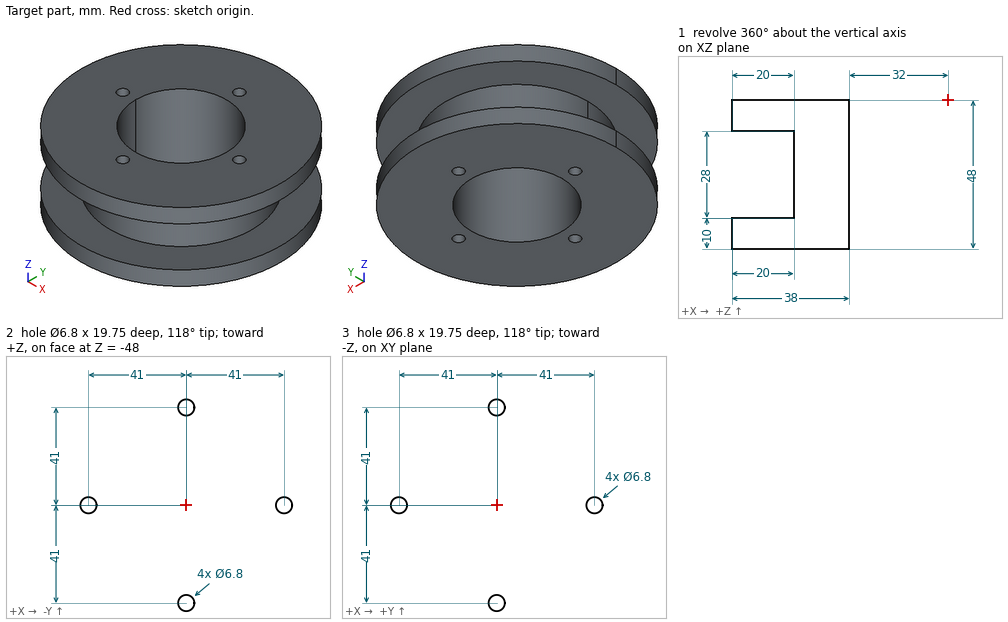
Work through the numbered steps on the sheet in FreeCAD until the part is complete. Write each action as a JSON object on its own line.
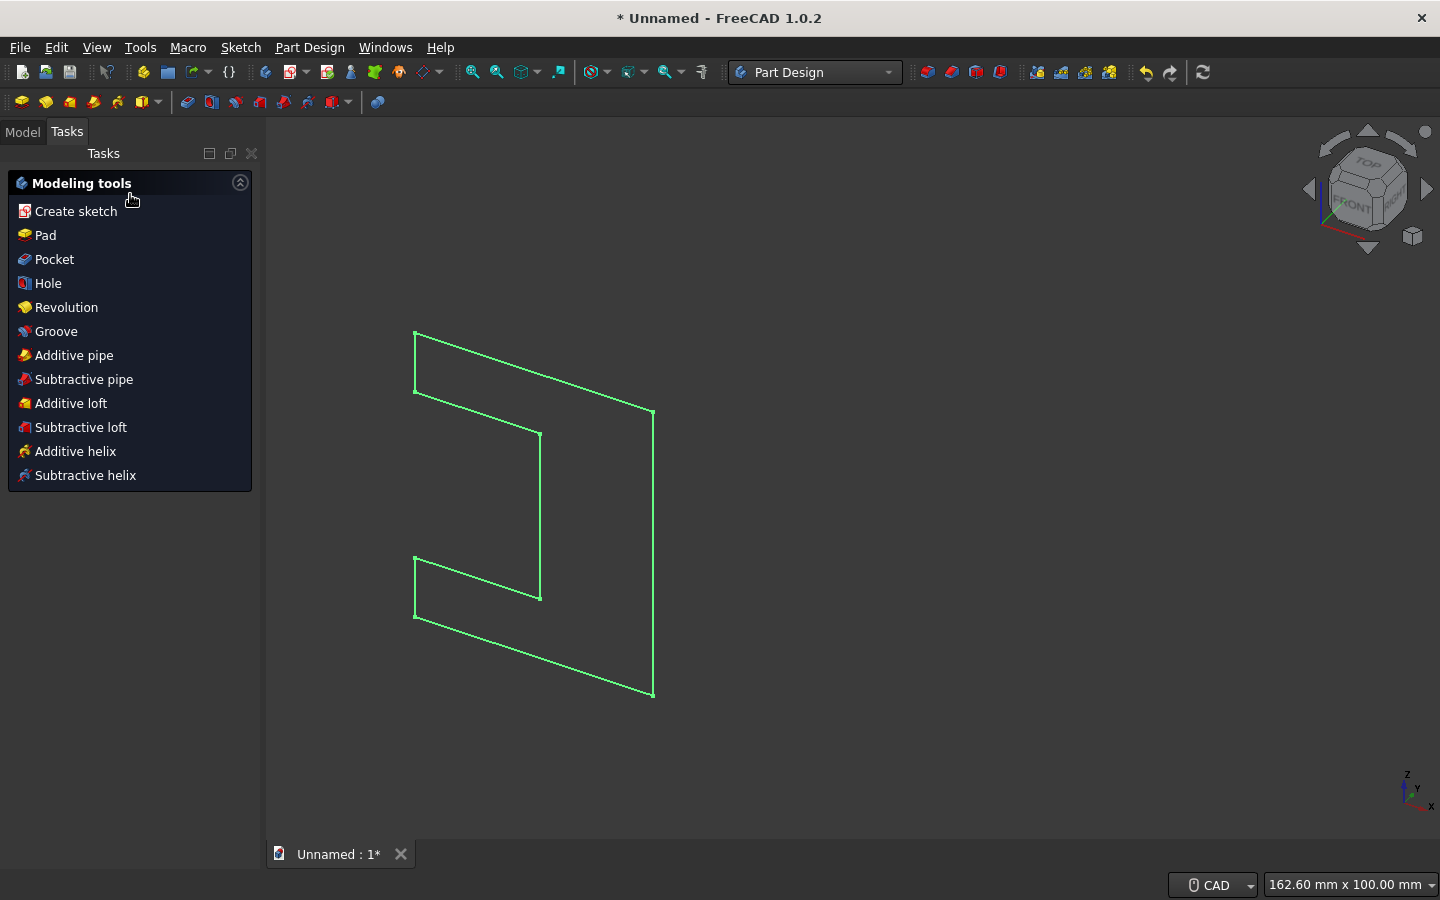
{"action": "left_click", "coordinate": [46, 102]}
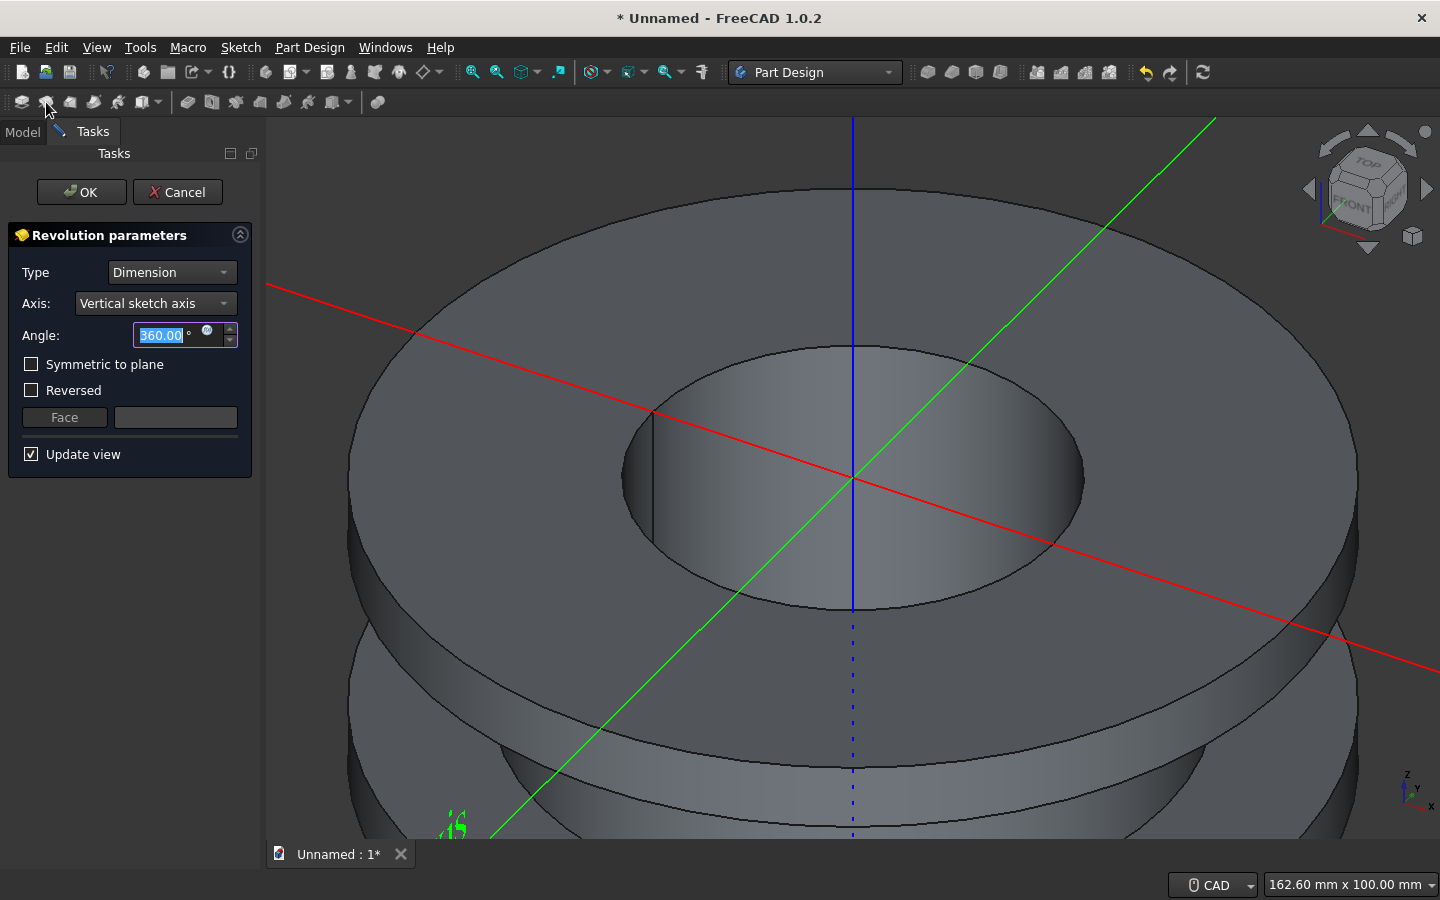
{"action": "left_click", "coordinate": [82, 192]}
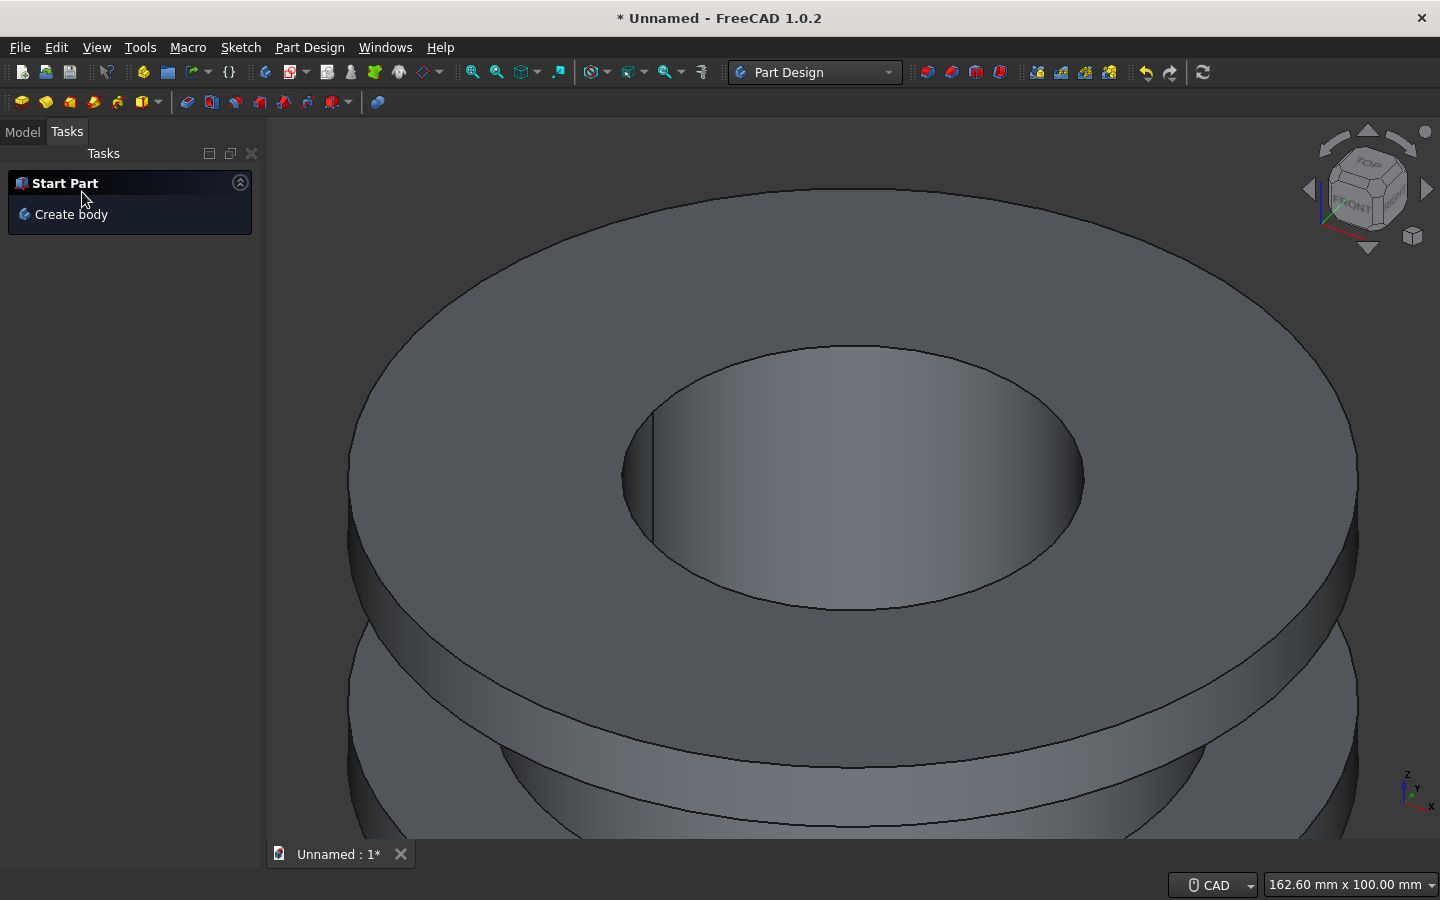
{"action": "left_click", "coordinate": [474, 72]}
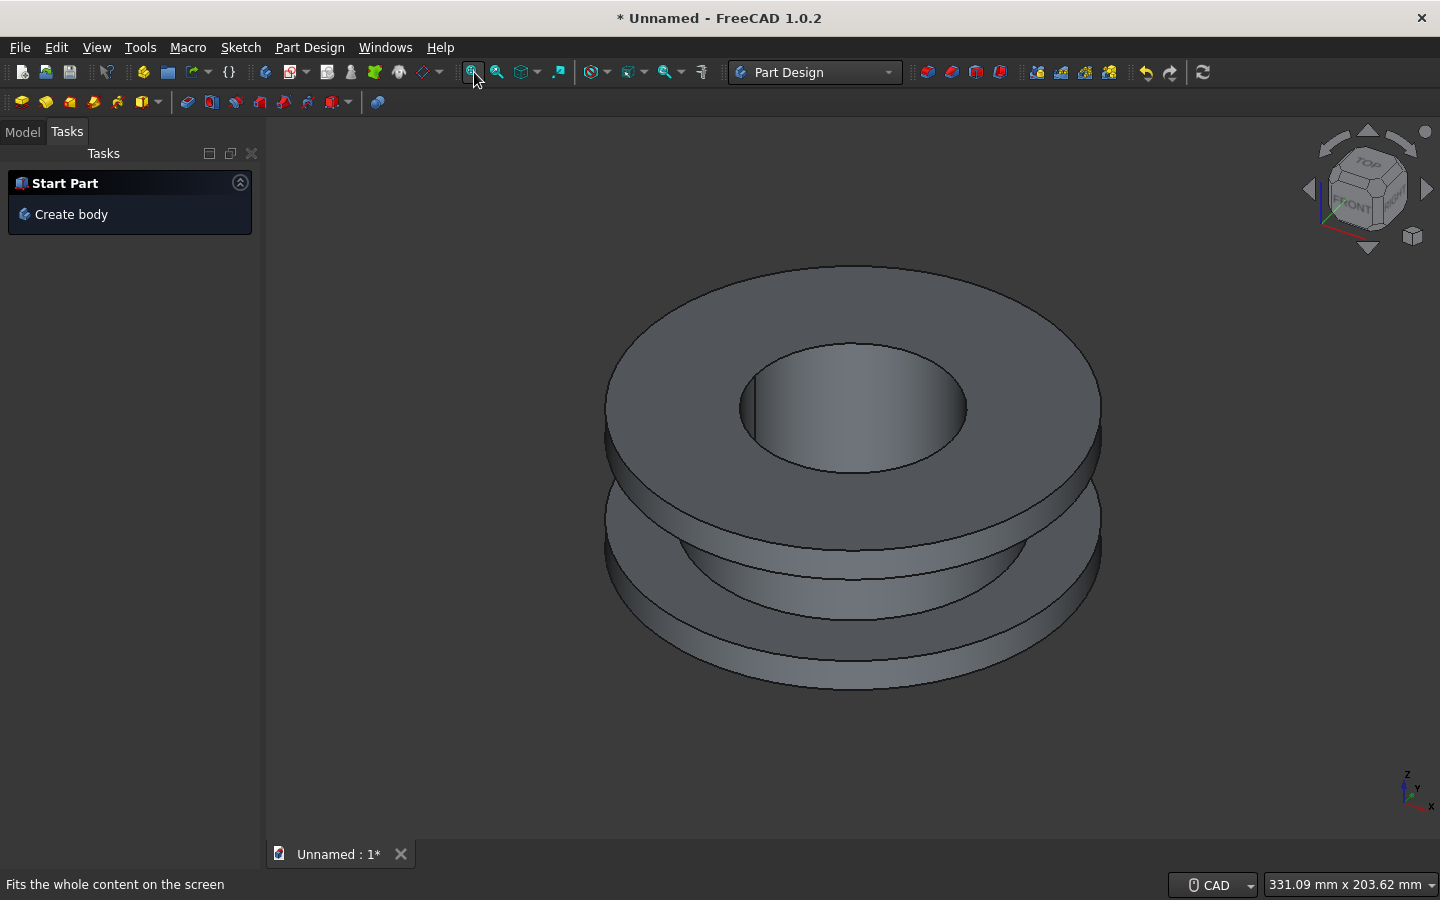
{"action": "key", "text": "5"}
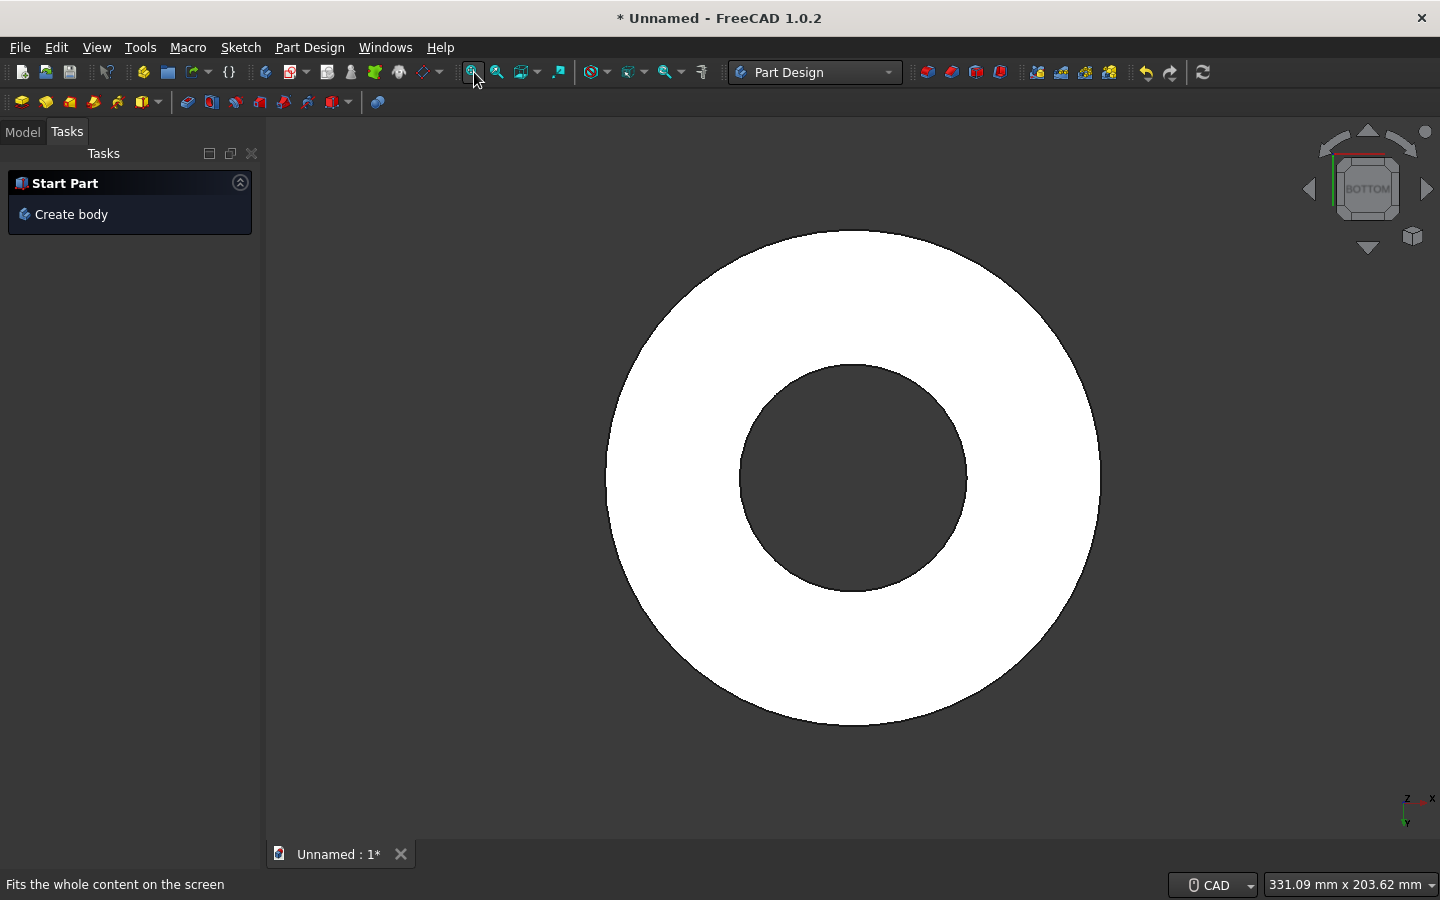
{"action": "left_click", "coordinate": [995, 619]}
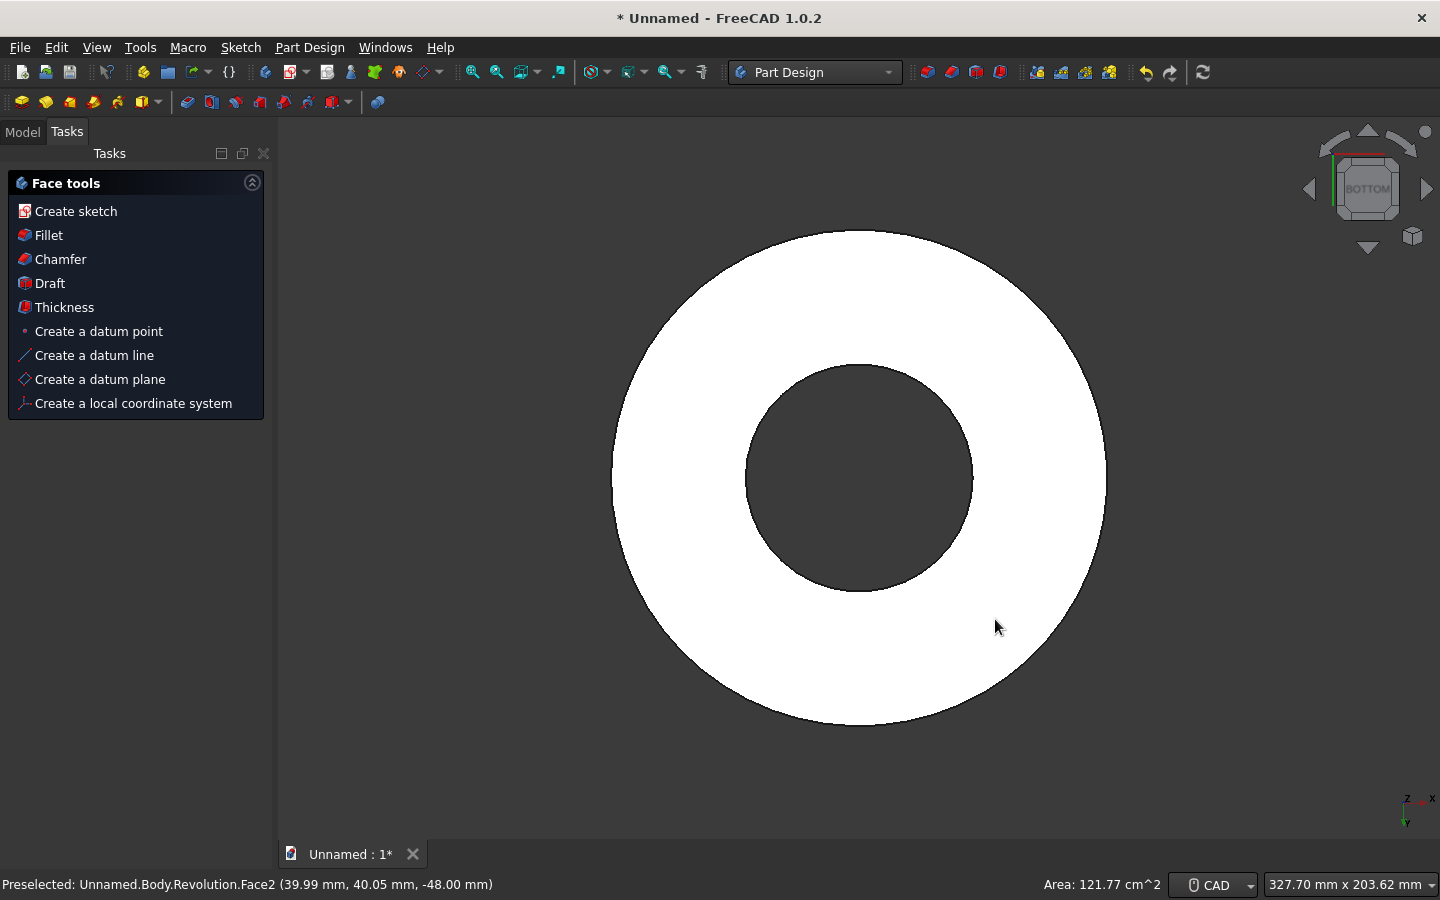
{"action": "left_click", "coordinate": [290, 72]}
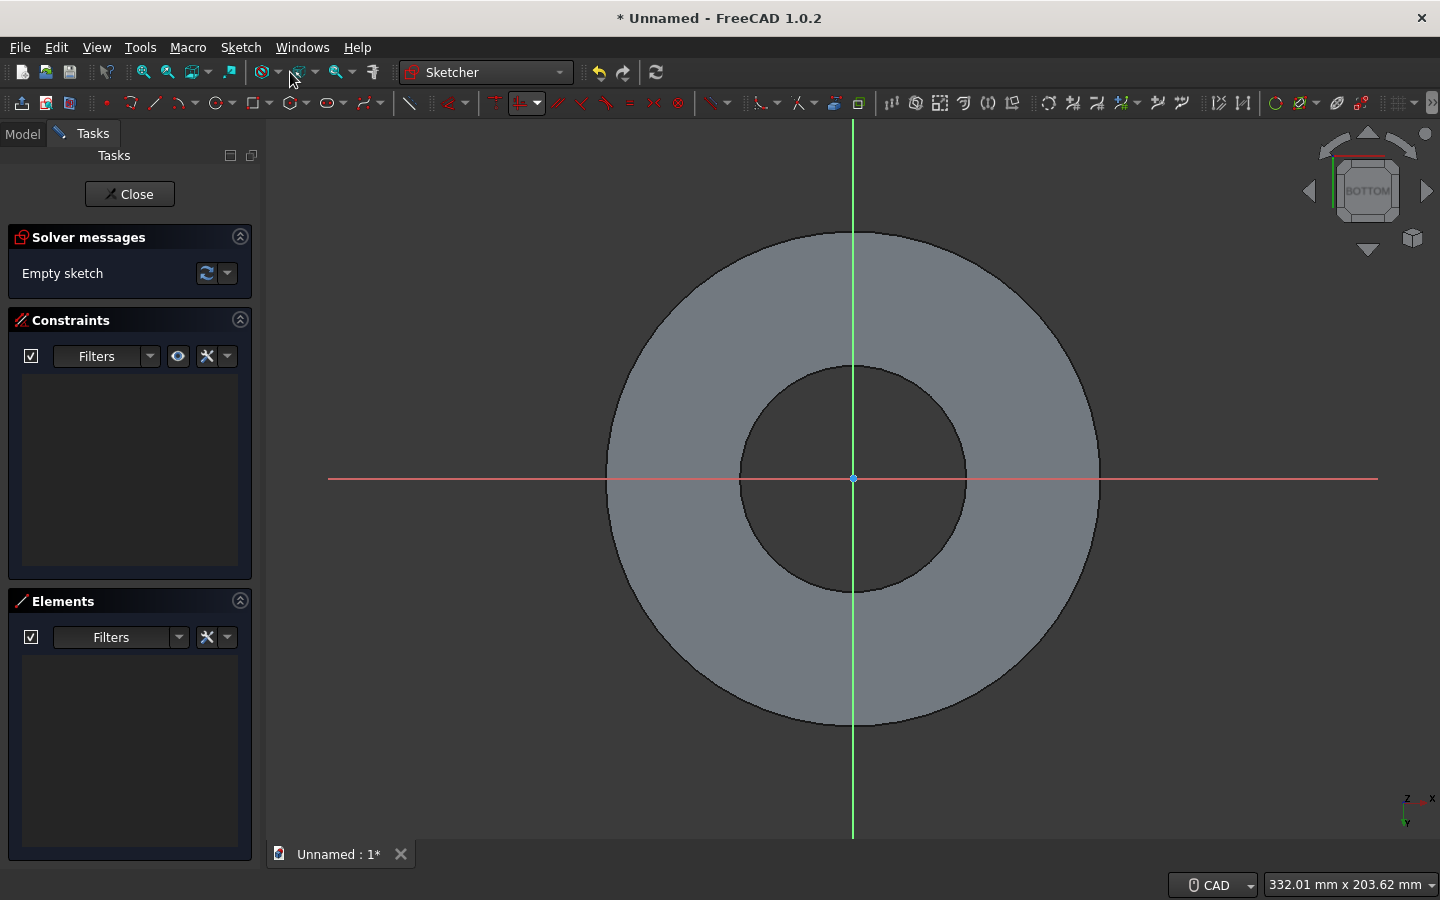
{"action": "scroll", "coordinate": [993, 479], "scroll_direction": "up", "scroll_amount": 2}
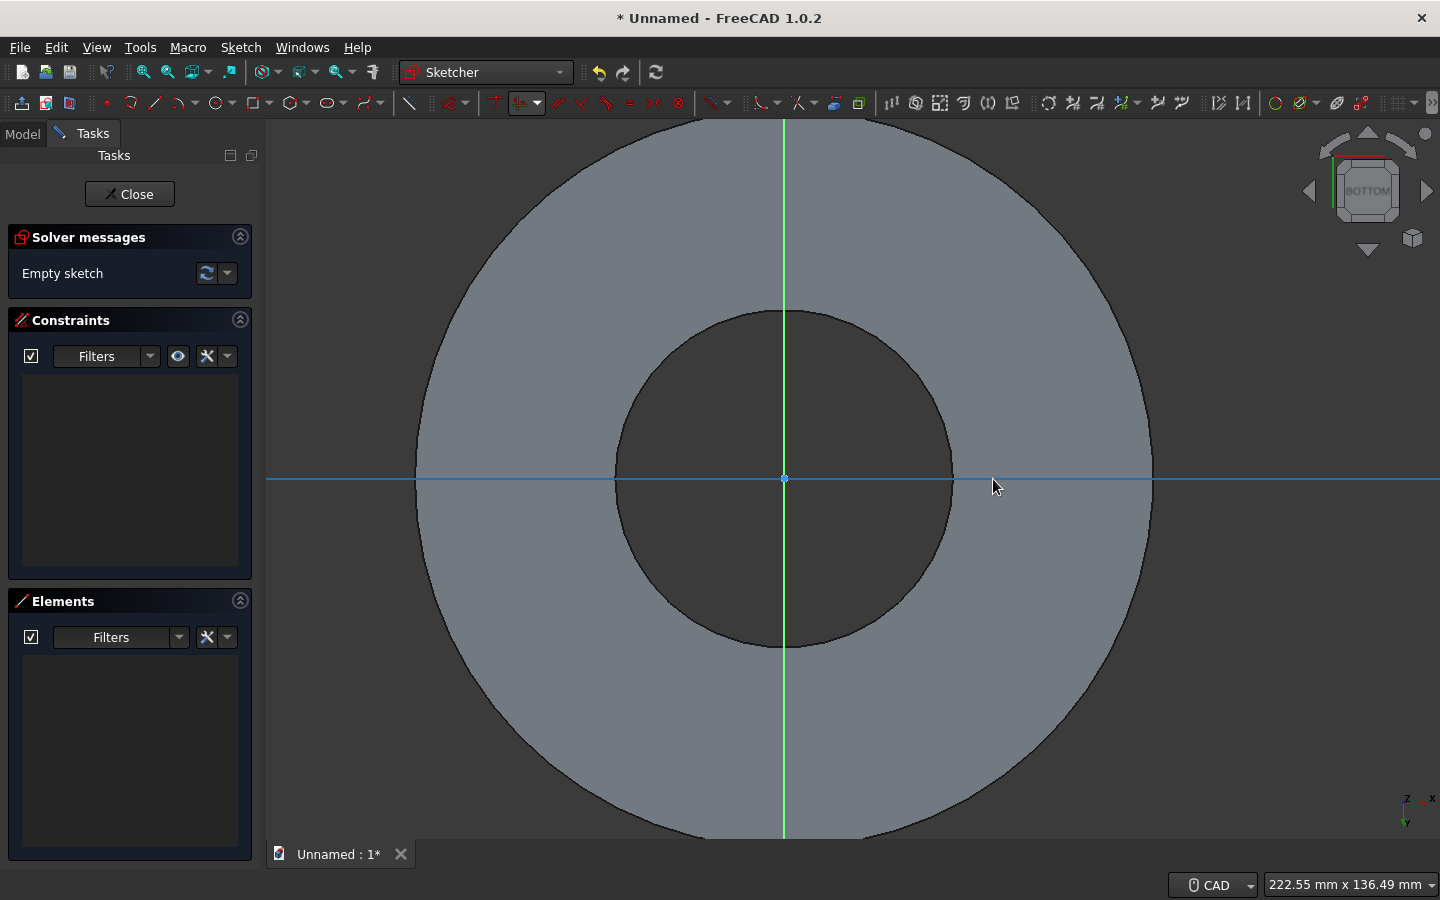
{"action": "left_click", "coordinate": [216, 104]}